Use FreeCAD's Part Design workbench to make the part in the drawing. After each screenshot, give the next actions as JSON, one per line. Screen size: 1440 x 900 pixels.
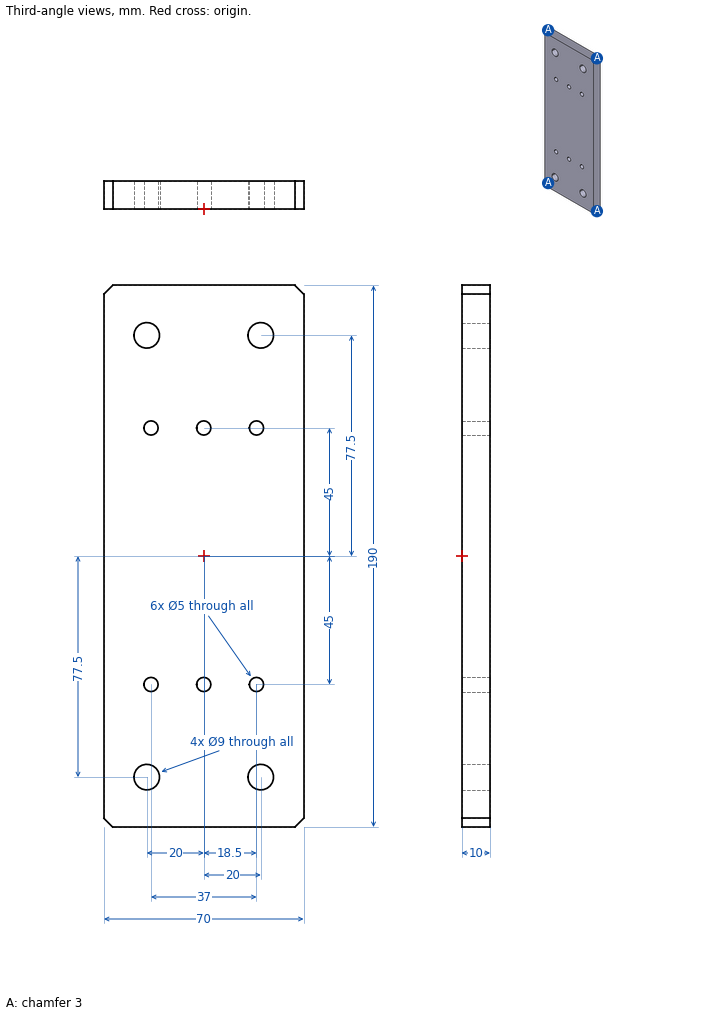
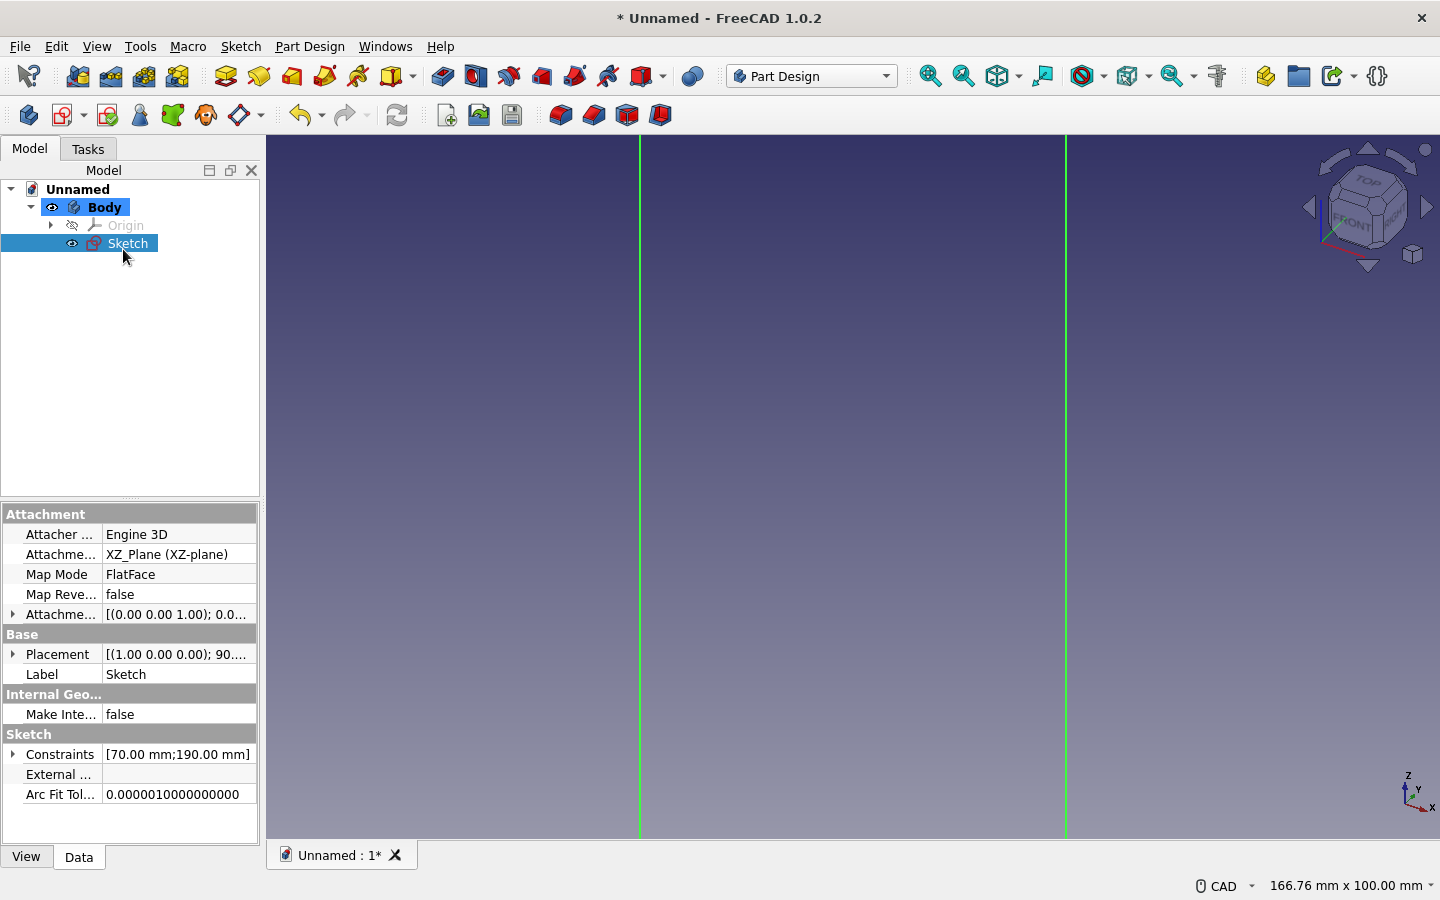
{"action": "left_click", "coordinate": [226, 76]}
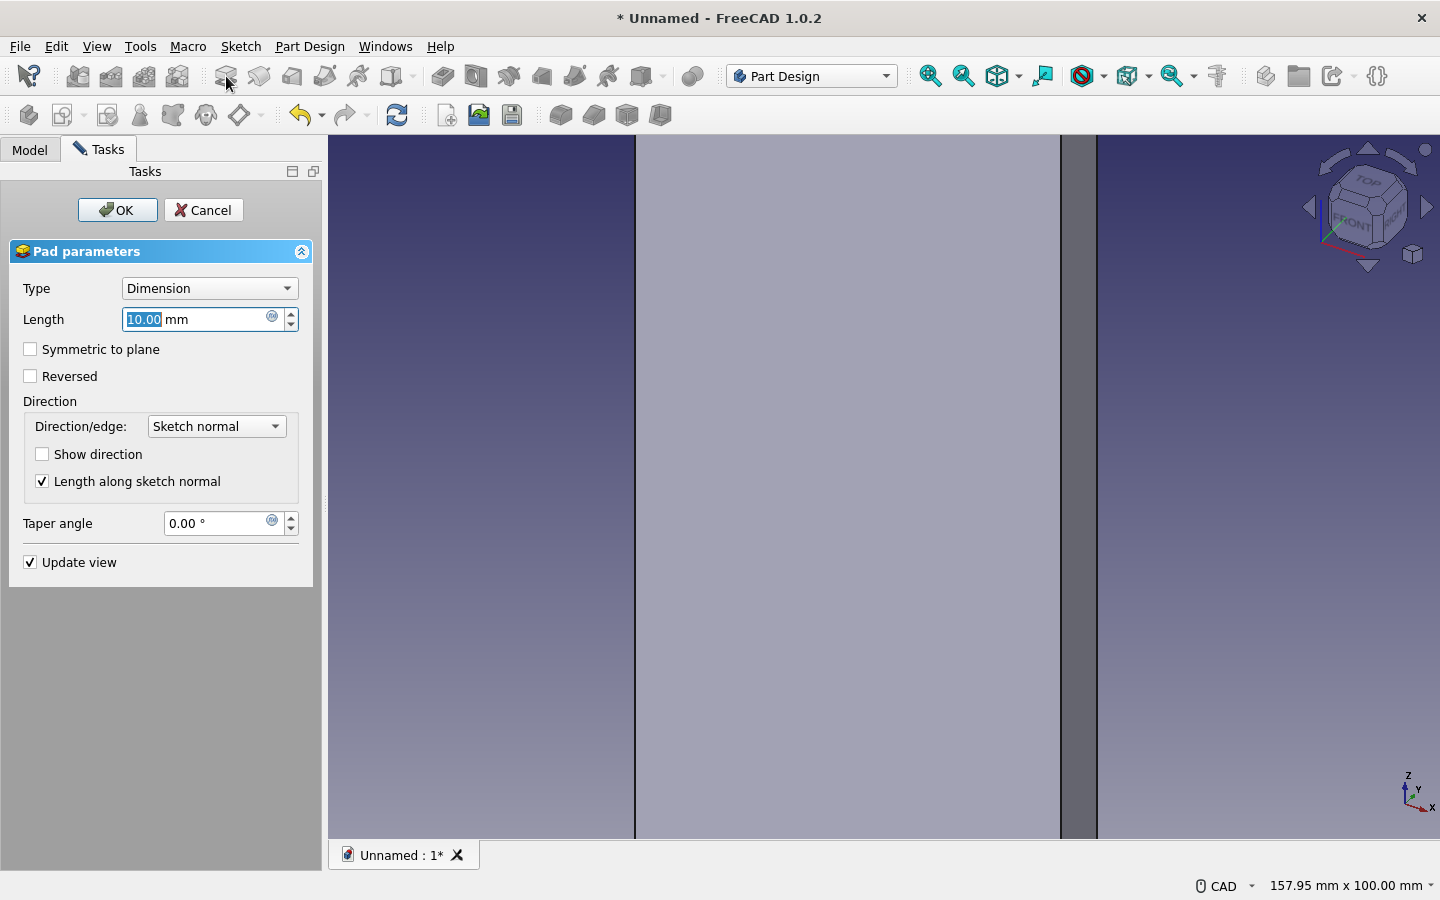
{"action": "type", "text": "10"}
{"action": "key", "text": "Tab"}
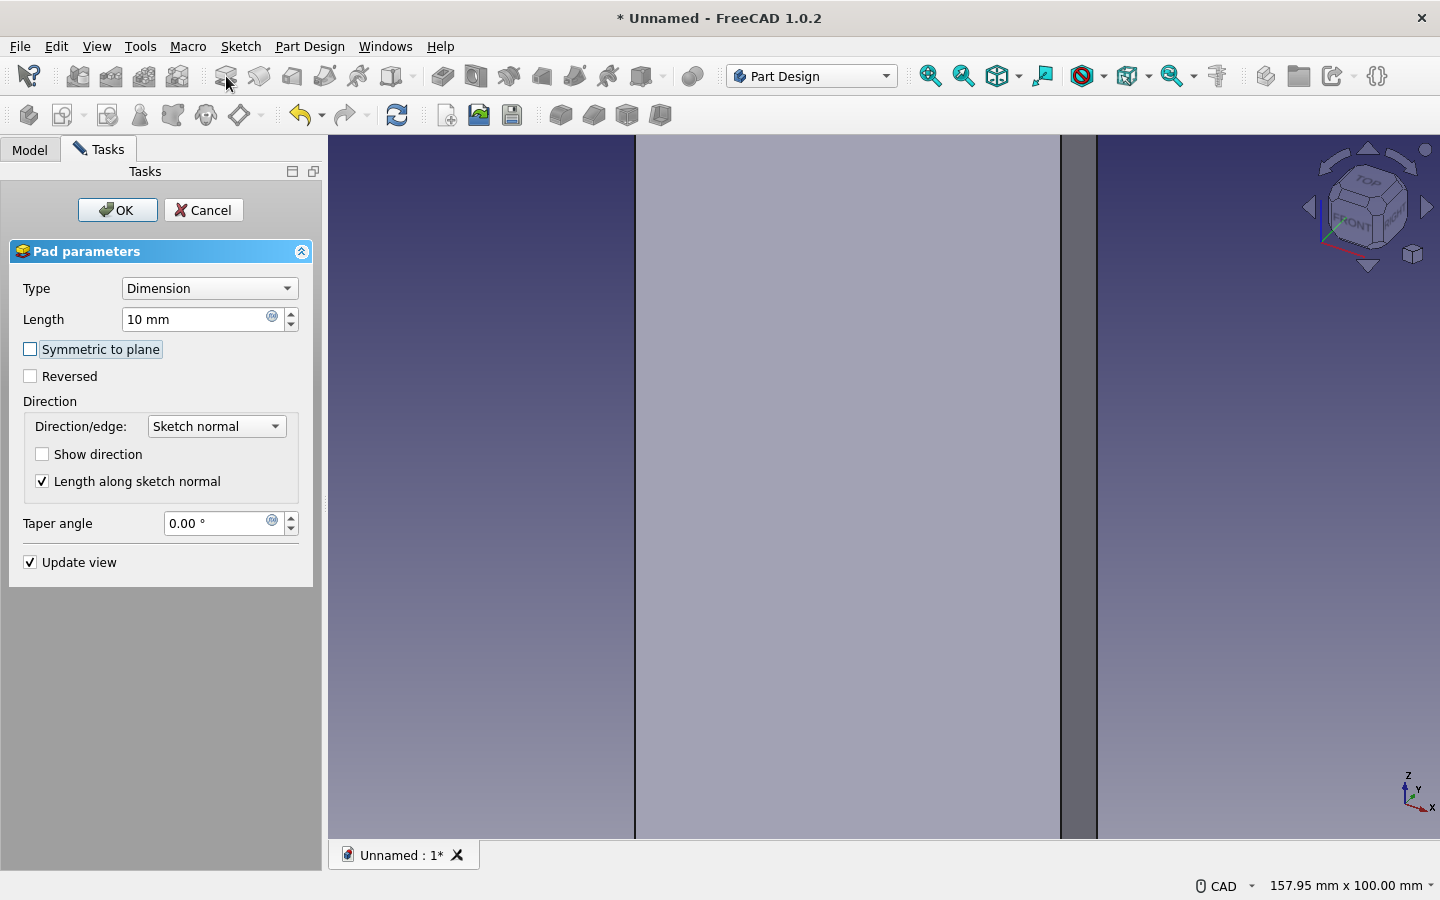
{"action": "left_click", "coordinate": [31, 376]}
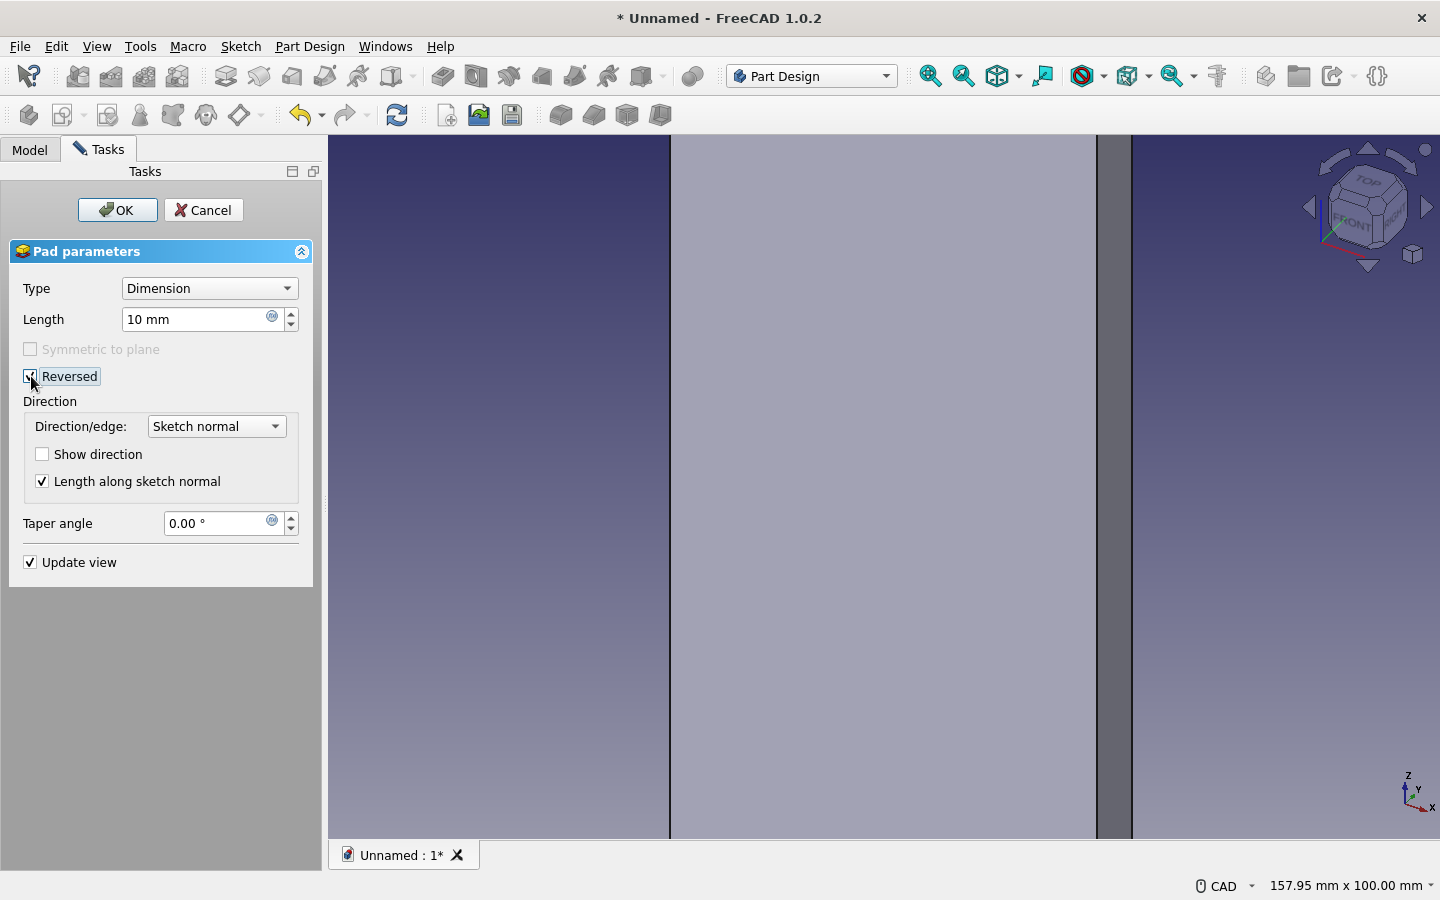
{"action": "left_click", "coordinate": [118, 210]}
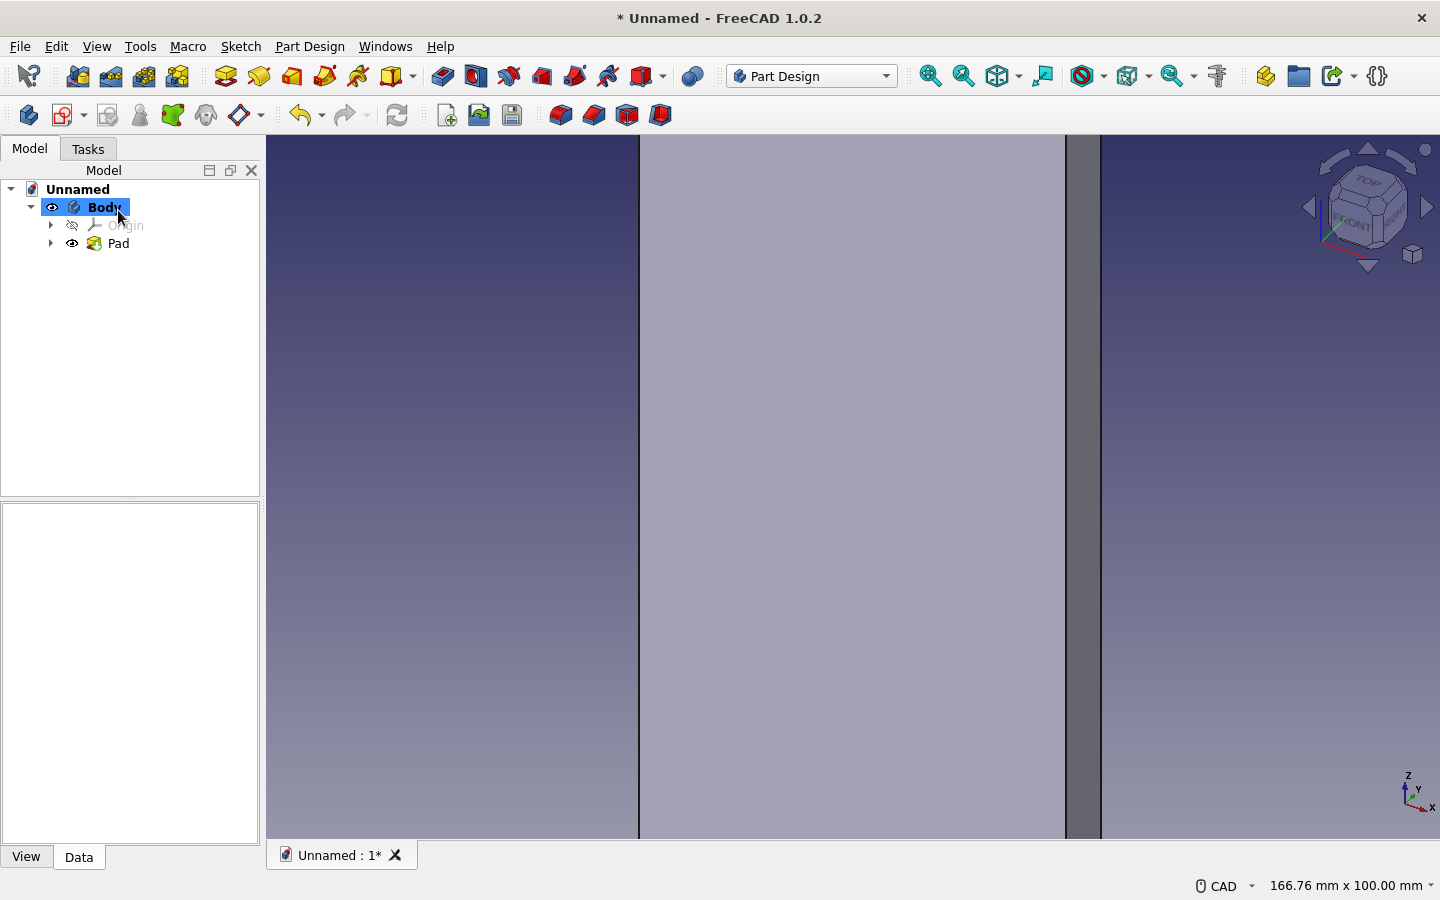
{"action": "left_click", "coordinate": [931, 76]}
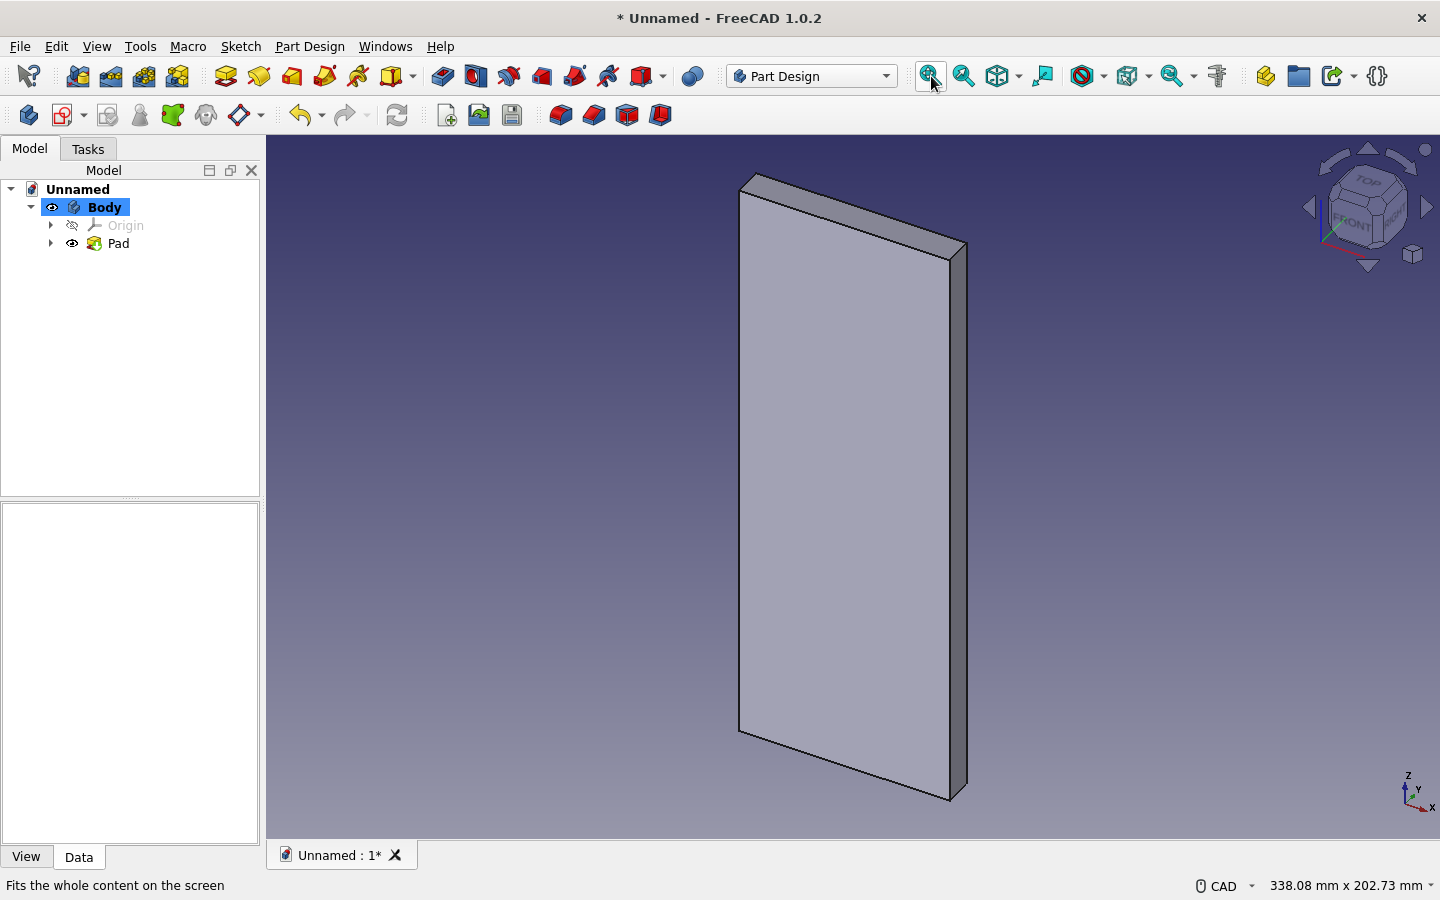
{"action": "key", "text": "4"}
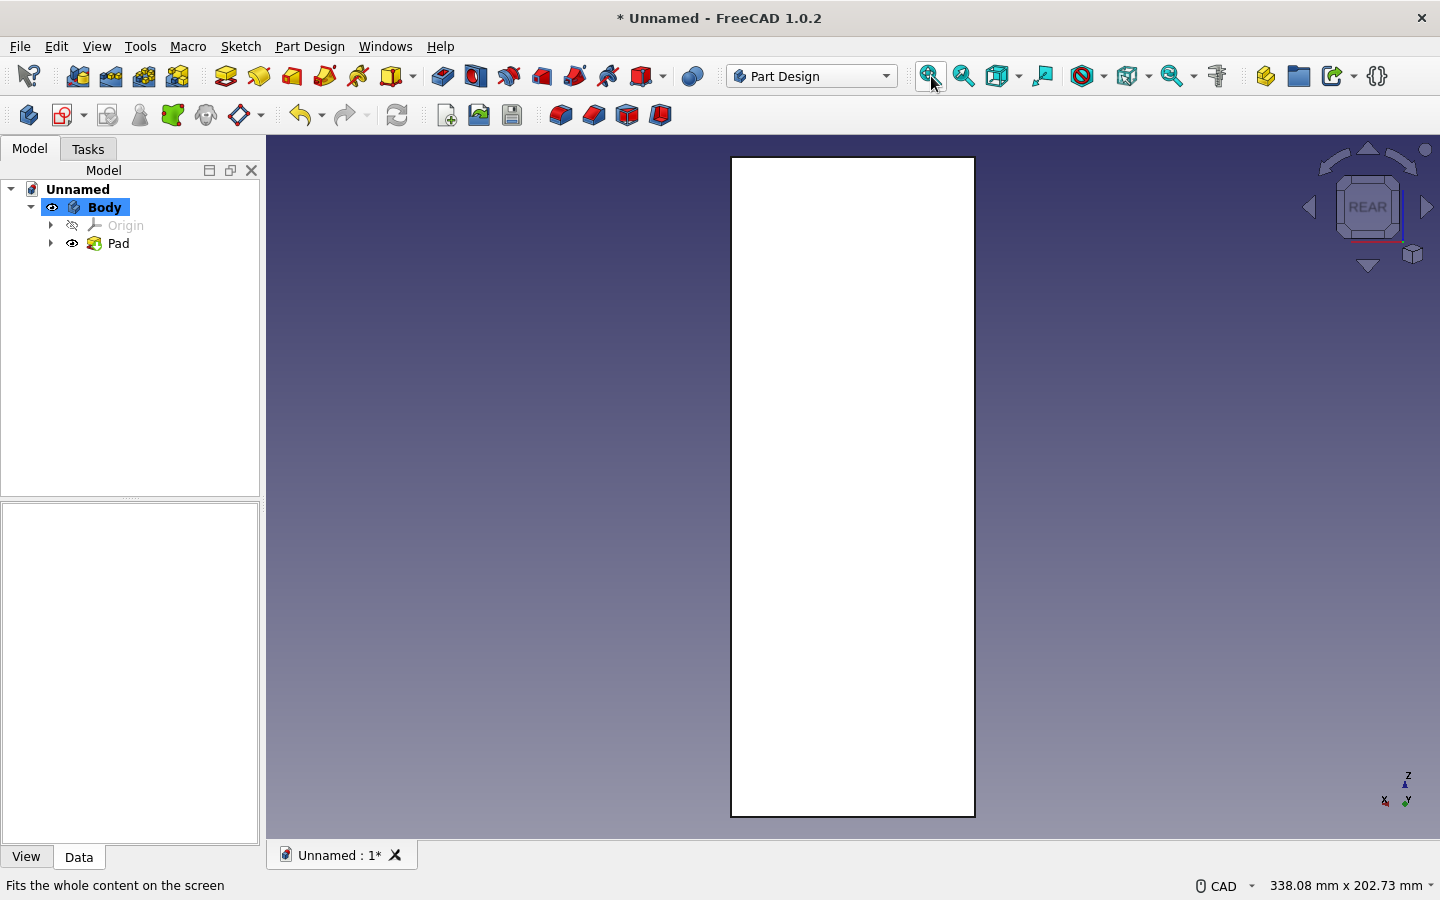
{"action": "left_click", "coordinate": [853, 297]}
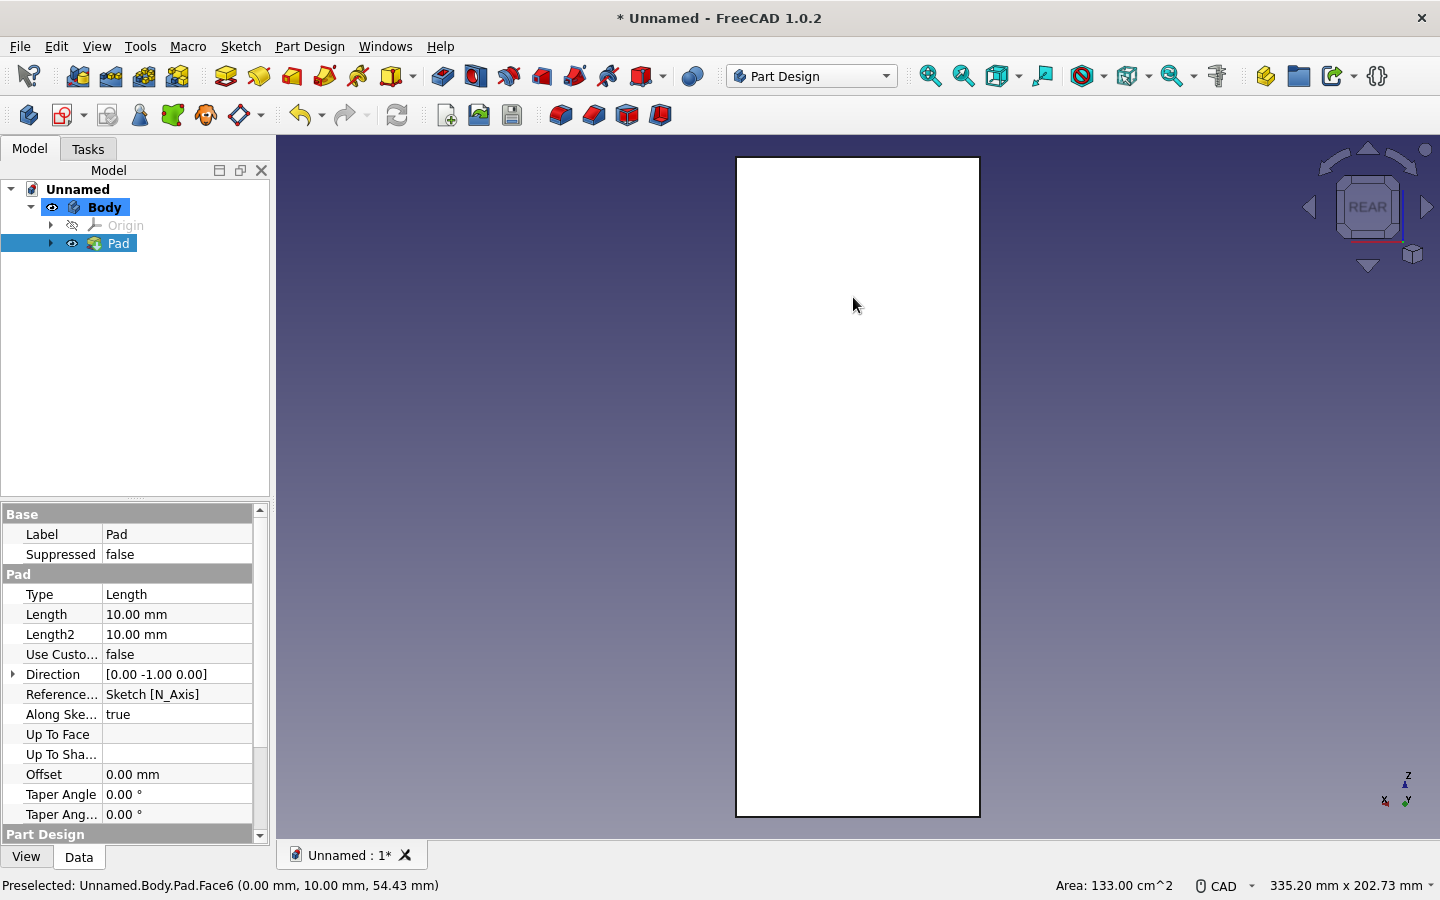
{"action": "left_click", "coordinate": [62, 116]}